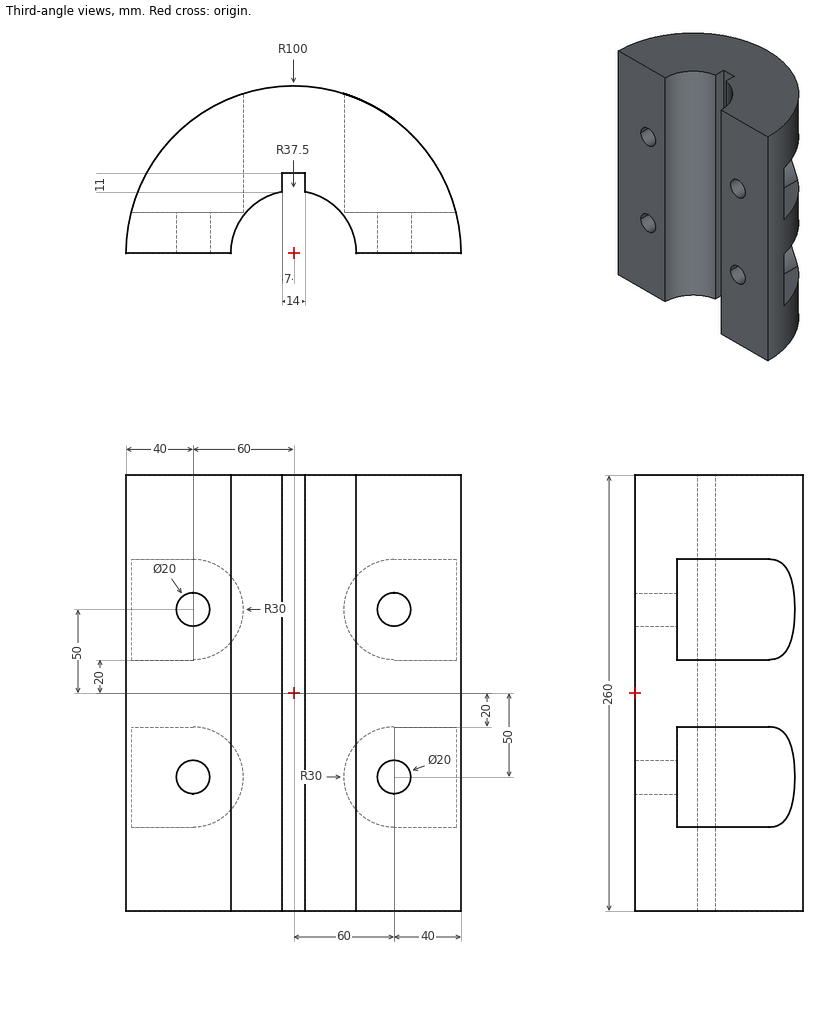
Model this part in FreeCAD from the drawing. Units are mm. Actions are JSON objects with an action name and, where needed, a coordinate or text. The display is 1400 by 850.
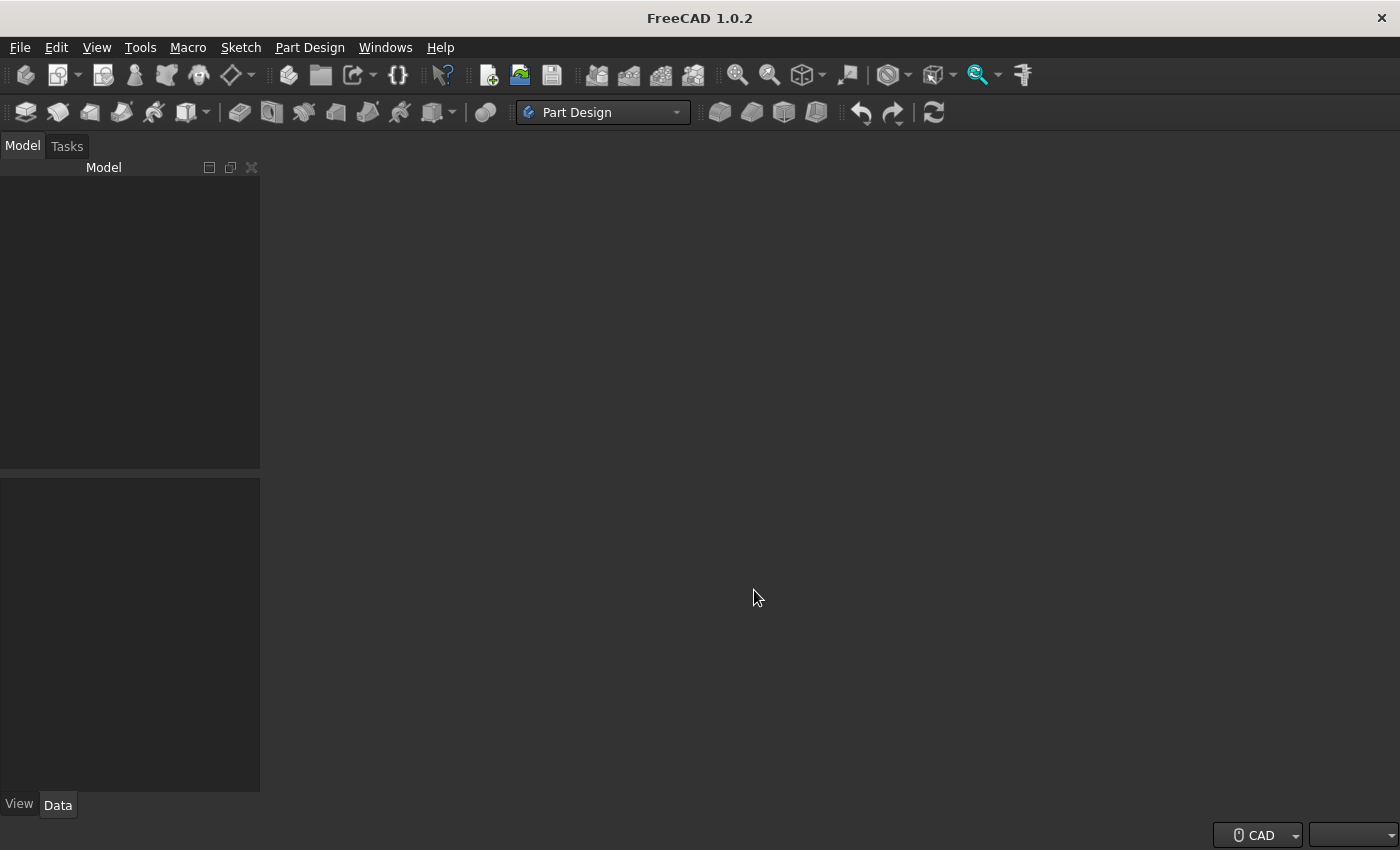
{"action": "left_click", "coordinate": [488, 76]}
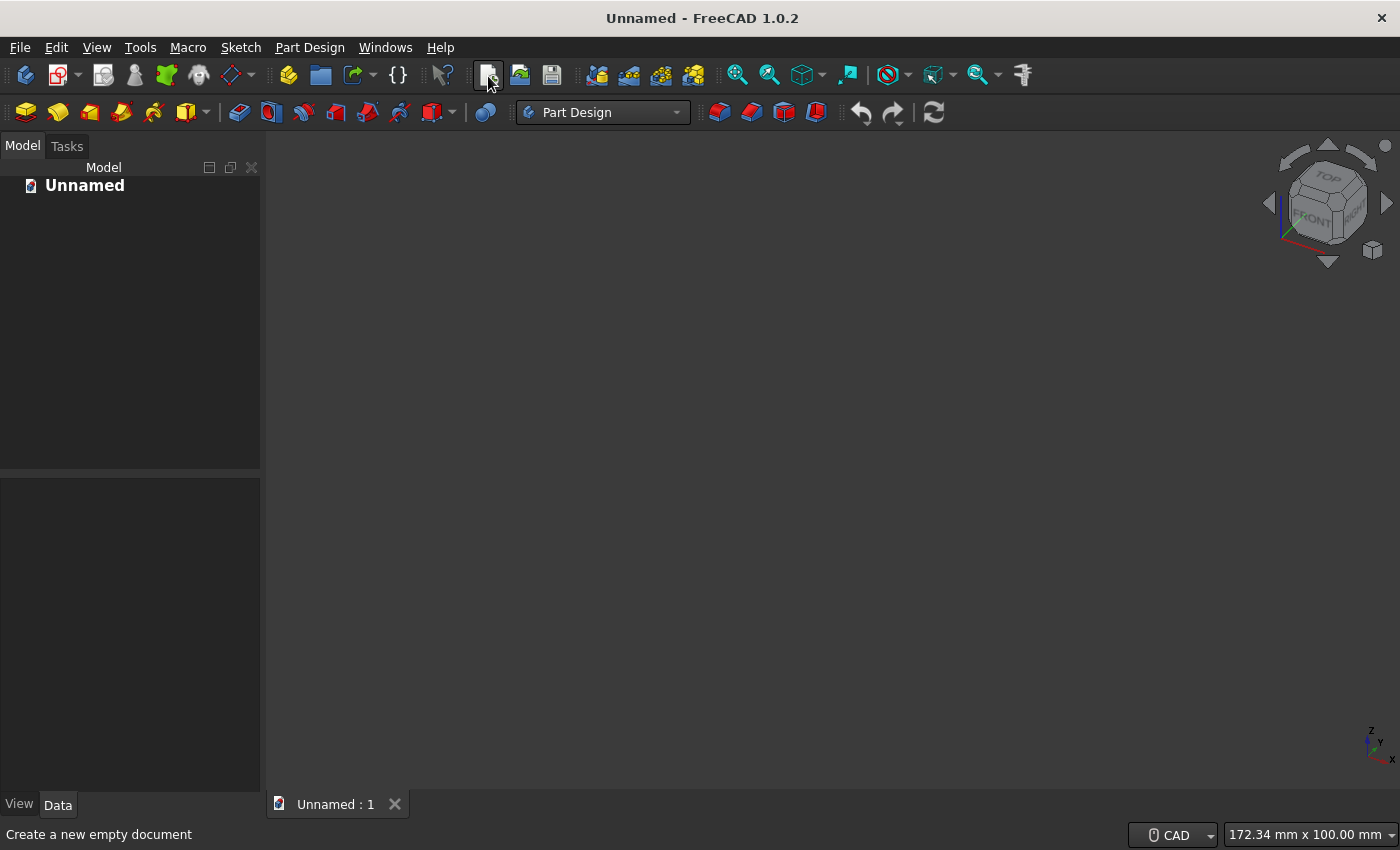
{"action": "left_click", "coordinate": [58, 76]}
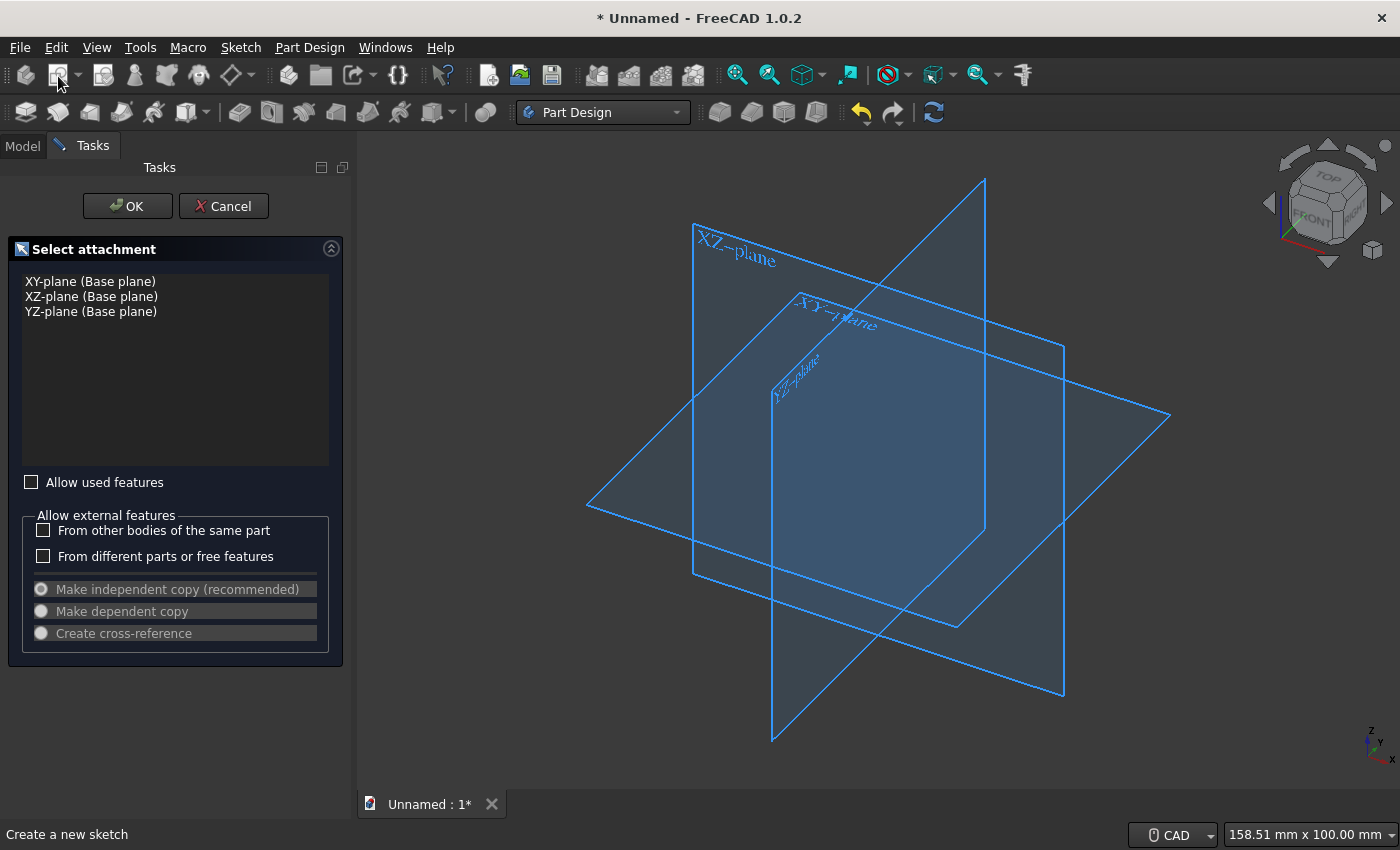
{"action": "left_click", "coordinate": [82, 282]}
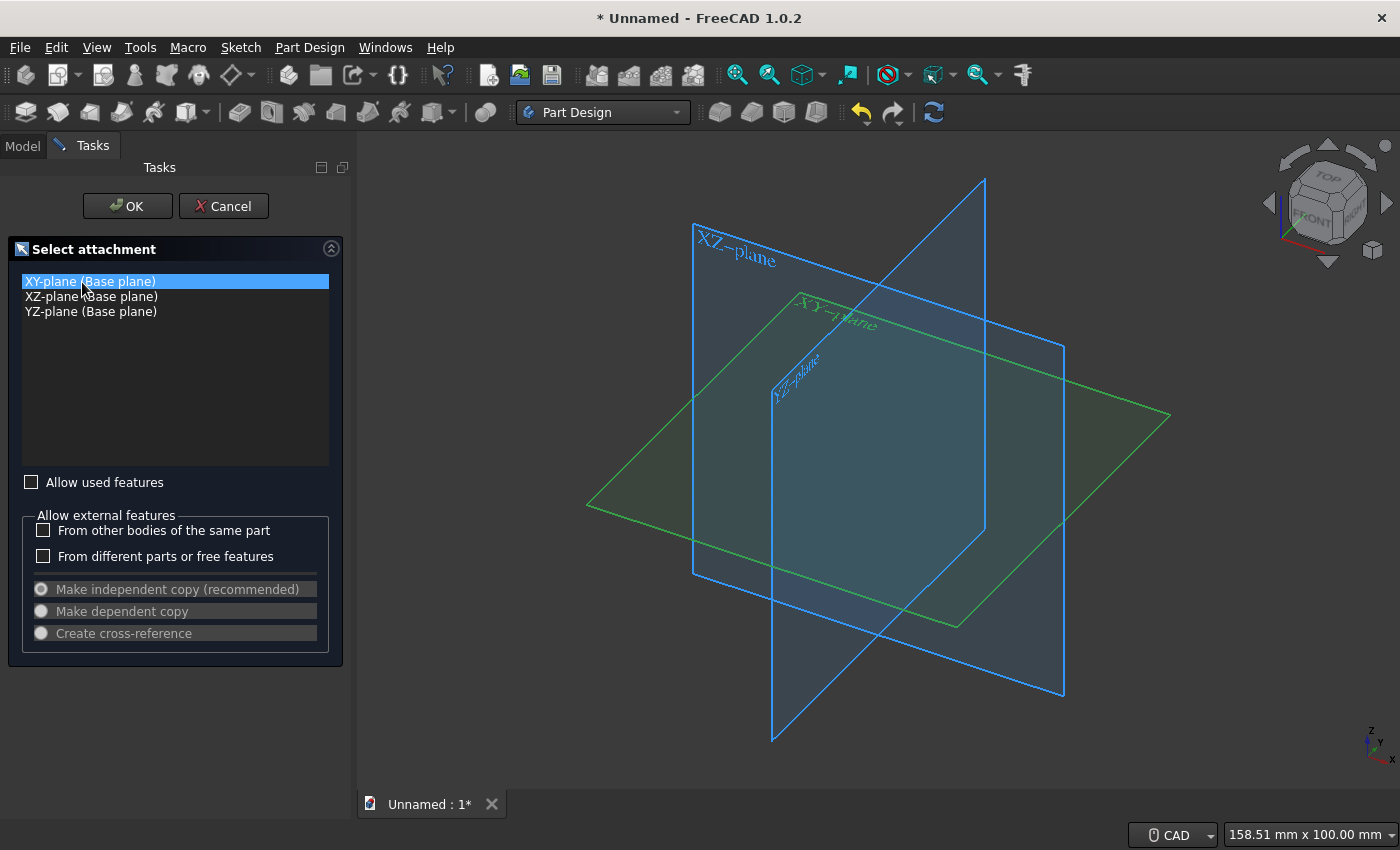
{"action": "left_click", "coordinate": [128, 206]}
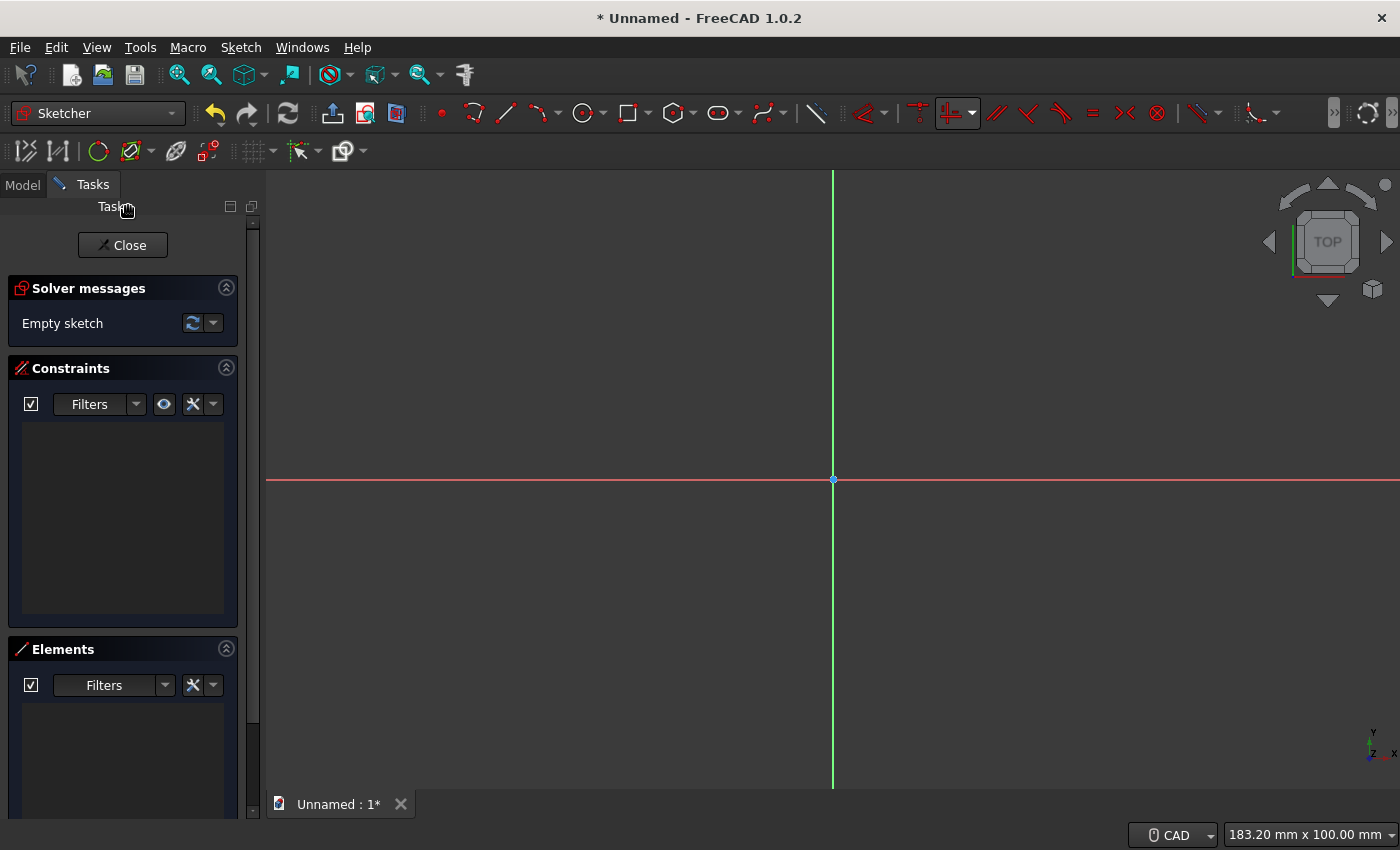
{"action": "scroll", "coordinate": [681, 761], "scroll_direction": "down", "scroll_amount": 3}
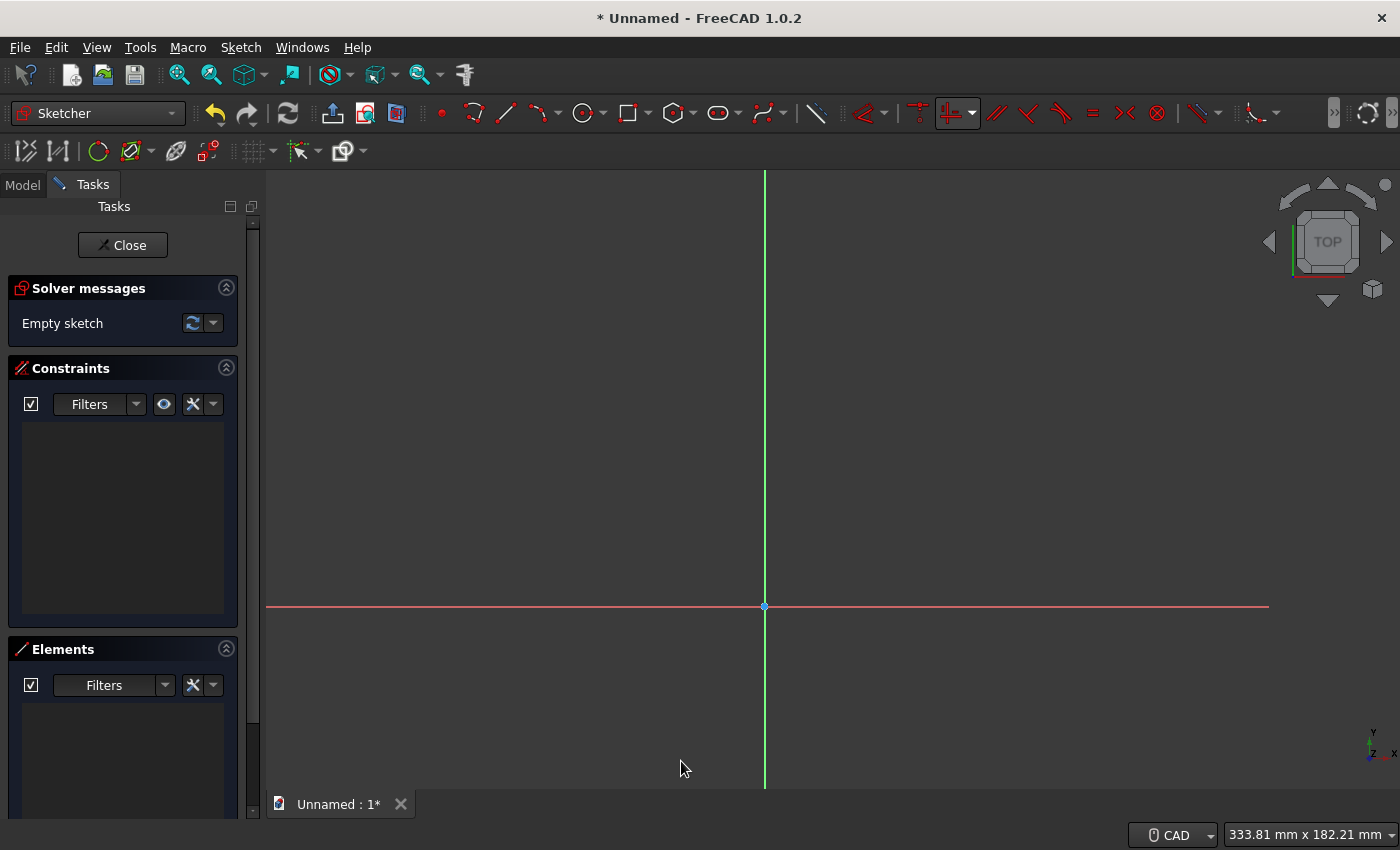
{"action": "left_click", "coordinate": [506, 114]}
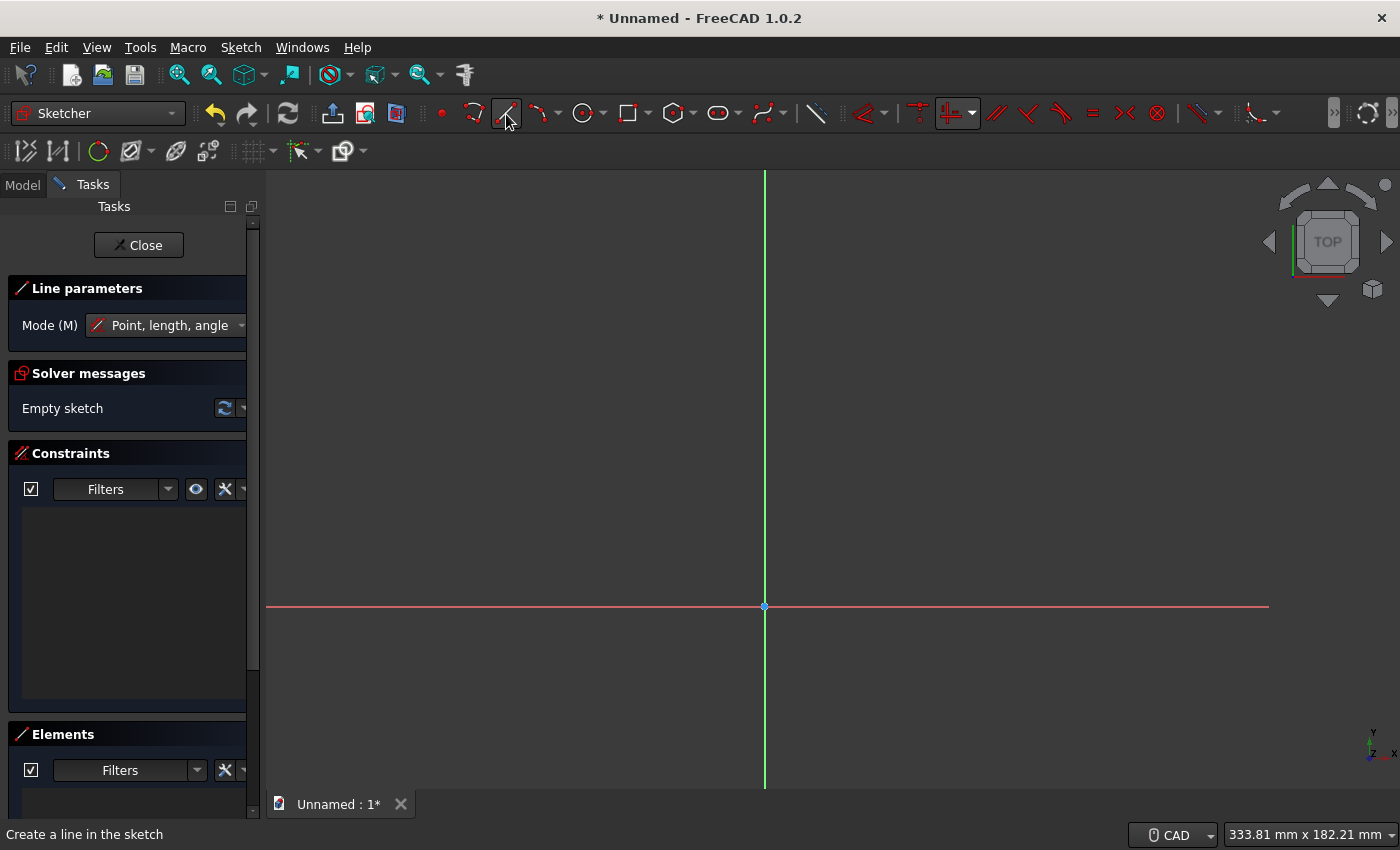
{"action": "left_click", "coordinate": [425, 607]}
{"action": "left_click", "coordinate": [637, 598]}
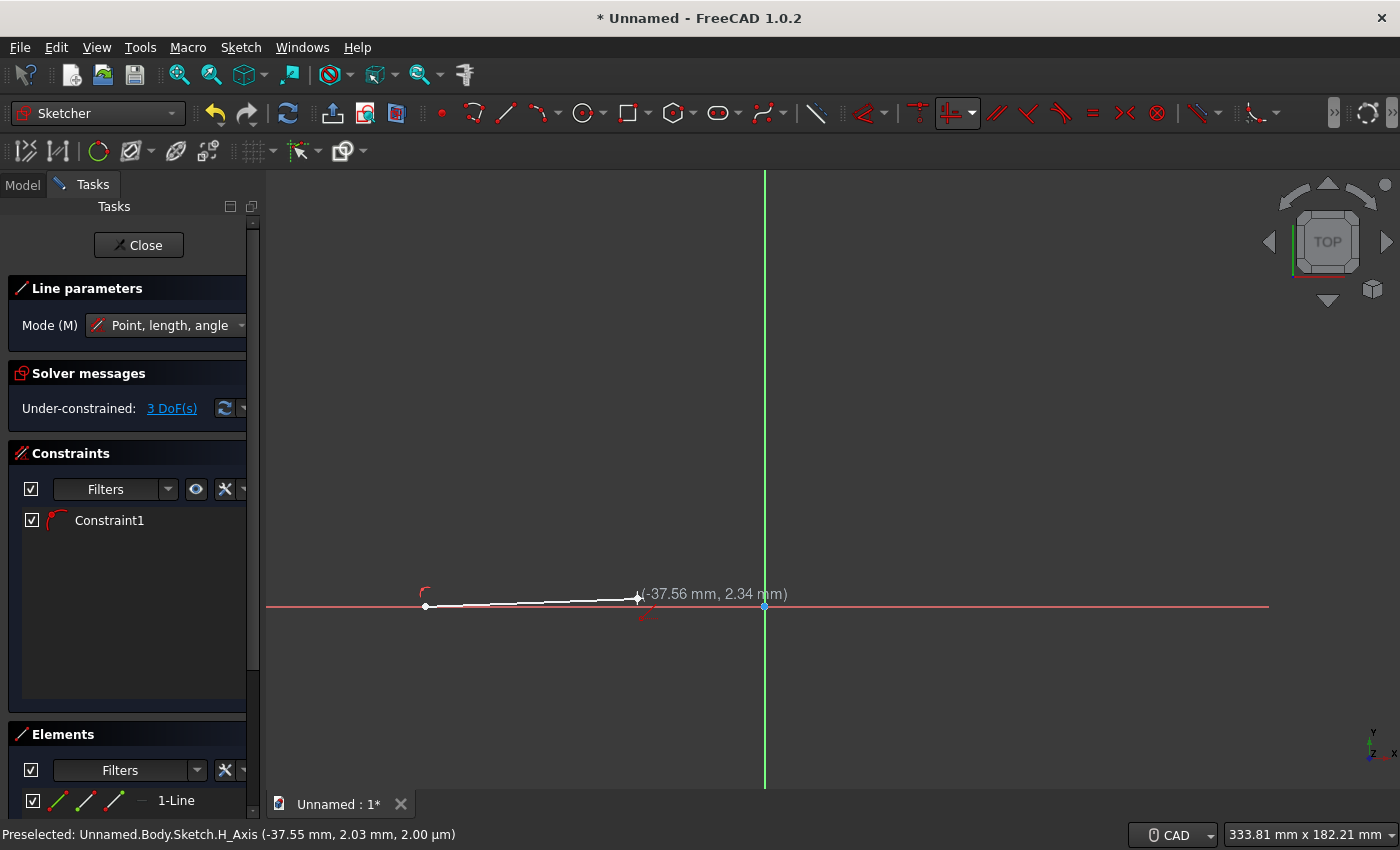
{"action": "left_click", "coordinate": [892, 607]}
{"action": "left_click", "coordinate": [1104, 598]}